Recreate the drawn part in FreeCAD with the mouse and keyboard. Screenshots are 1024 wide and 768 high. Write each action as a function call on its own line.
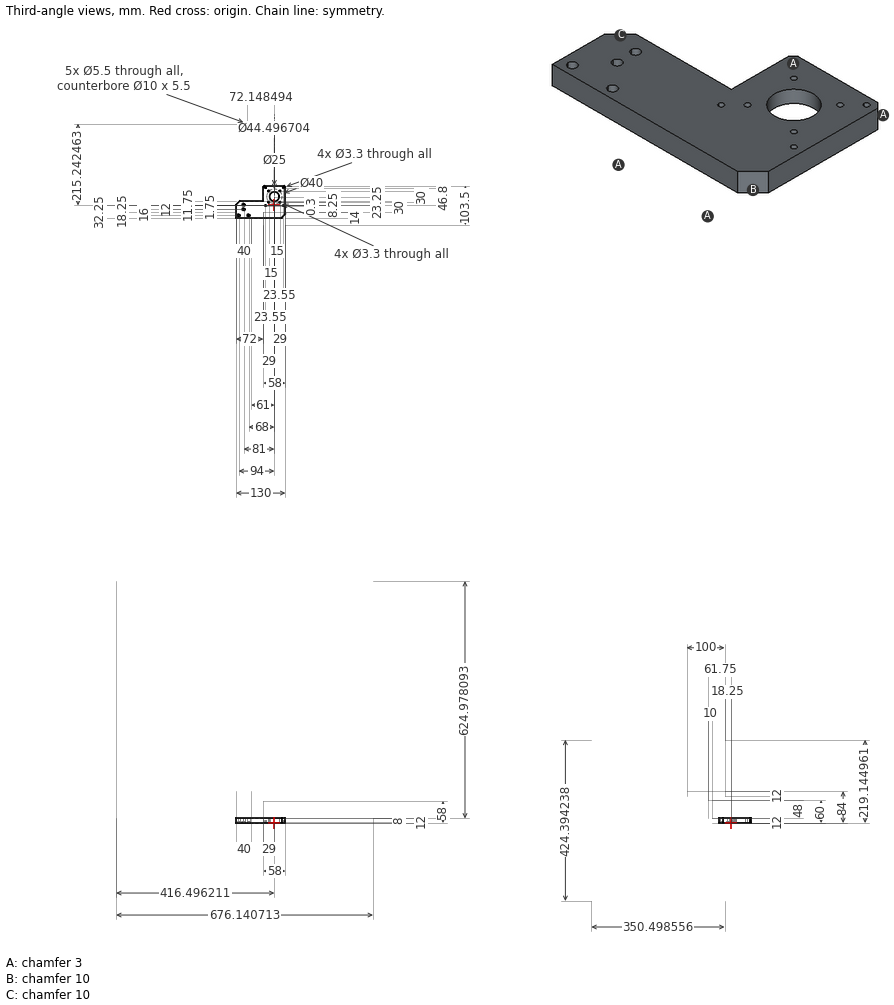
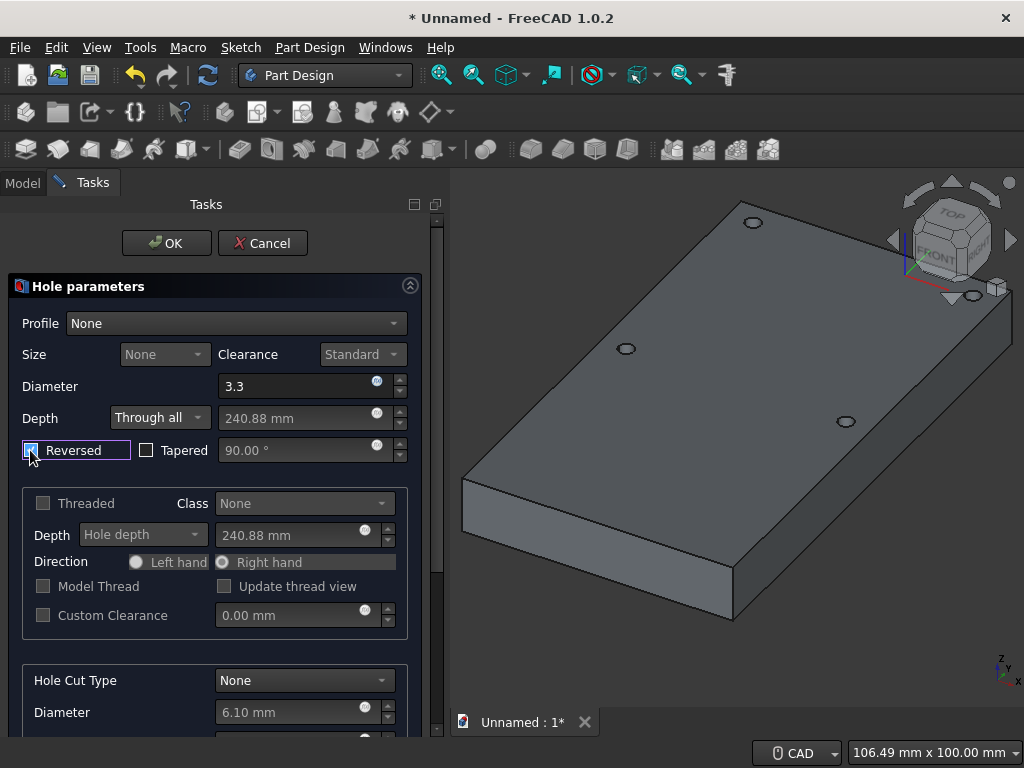
click(167, 243)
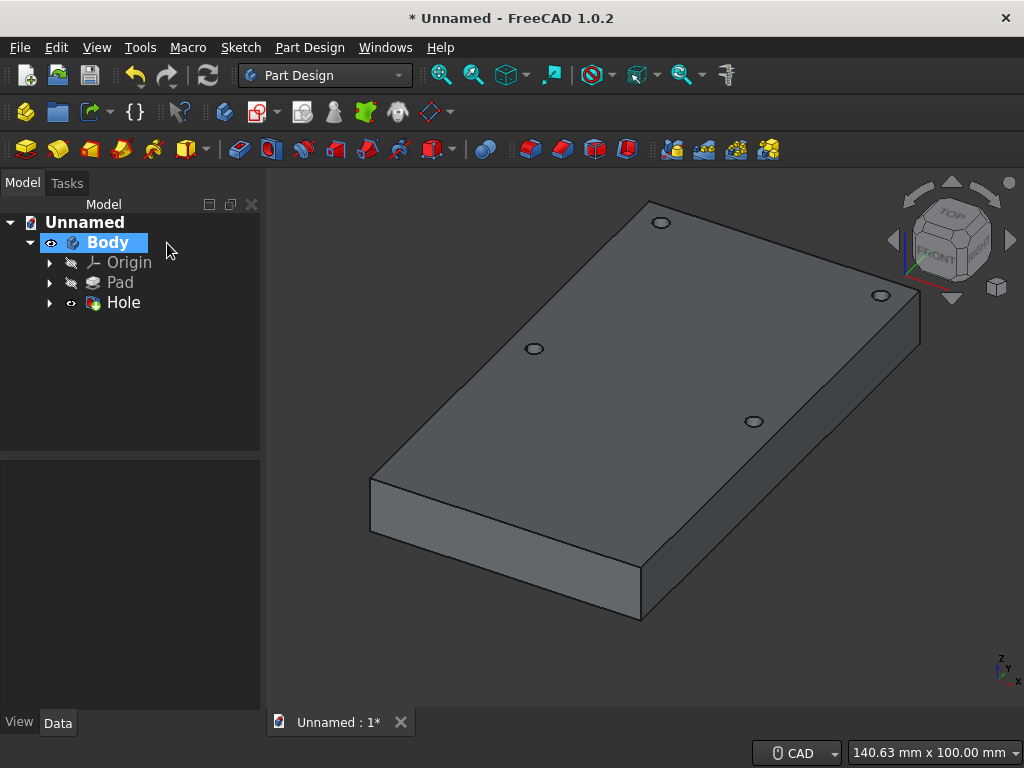
key(5)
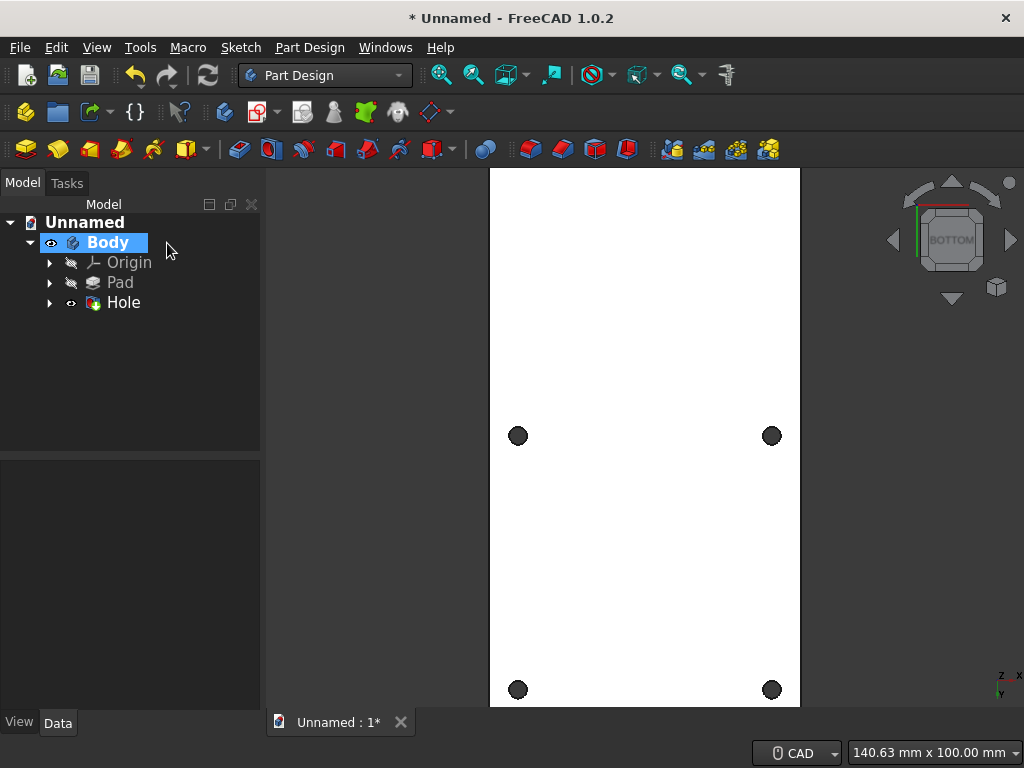
click(442, 76)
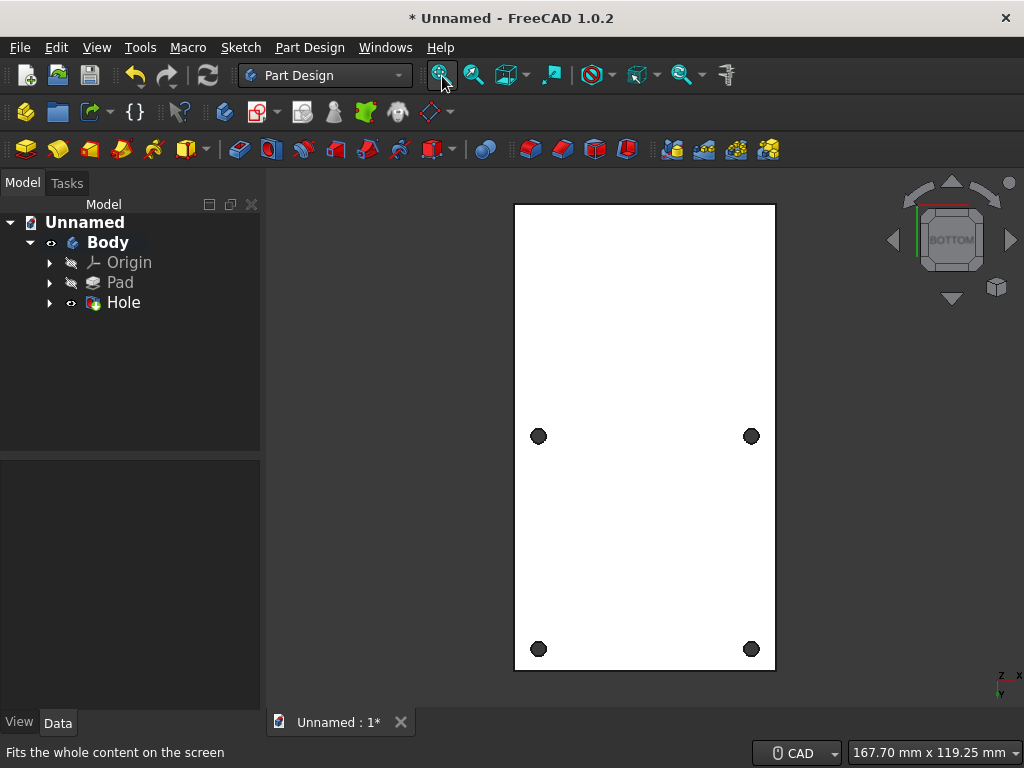
click(645, 503)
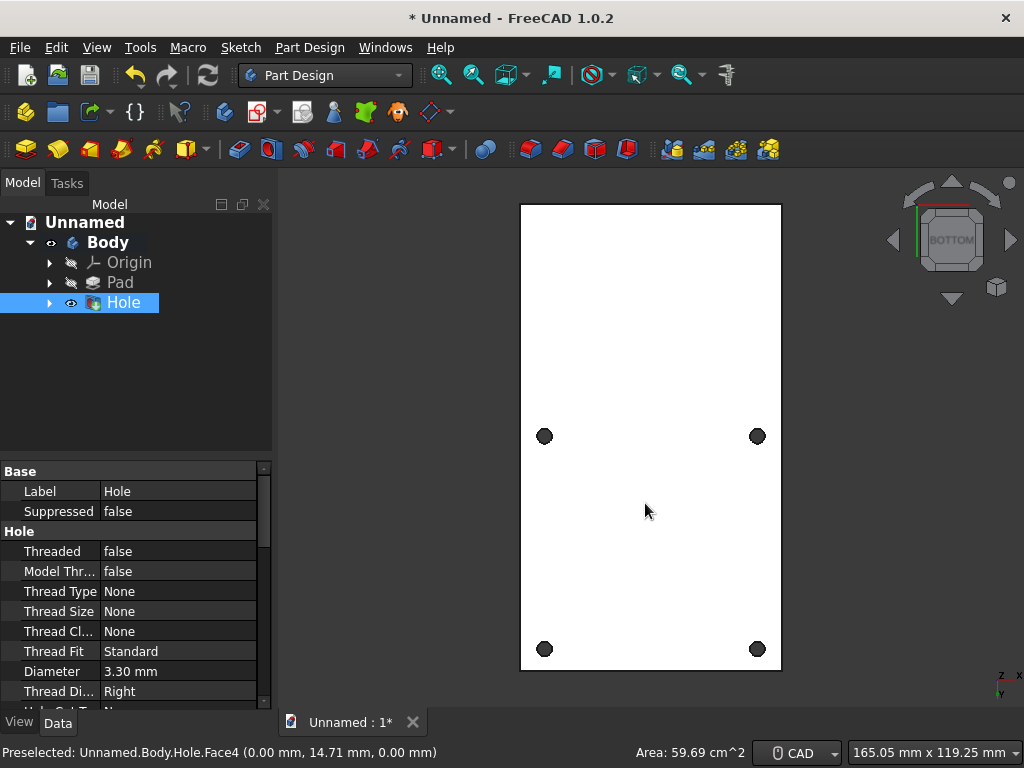
click(258, 112)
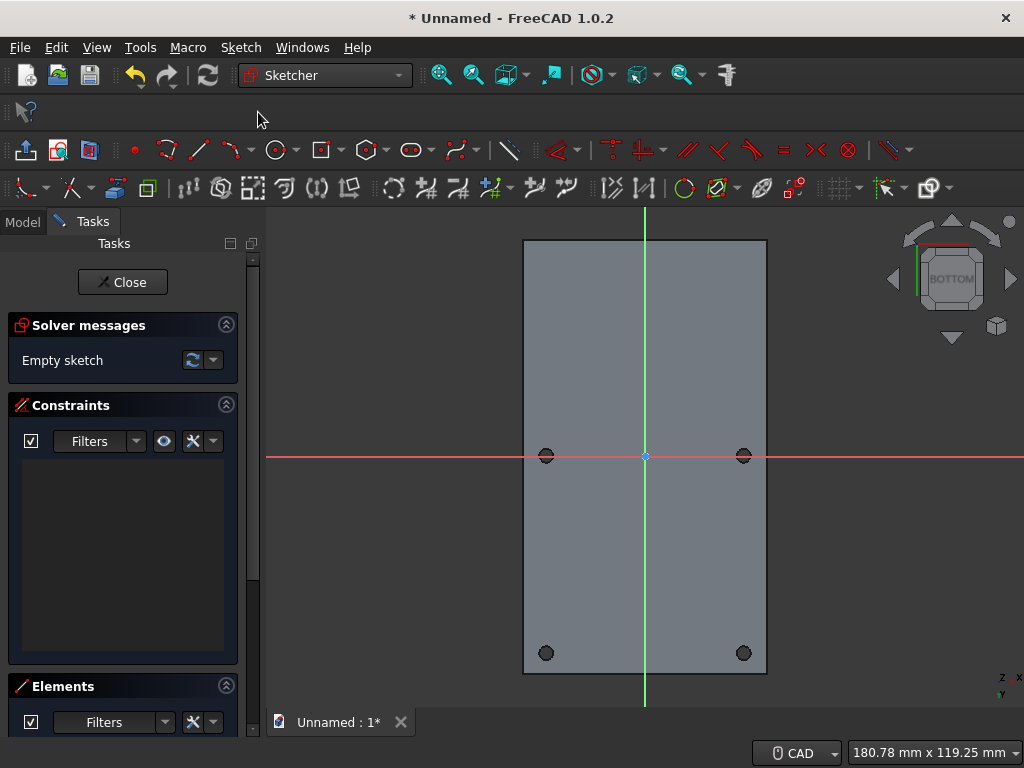
scroll(728, 658, up, 3)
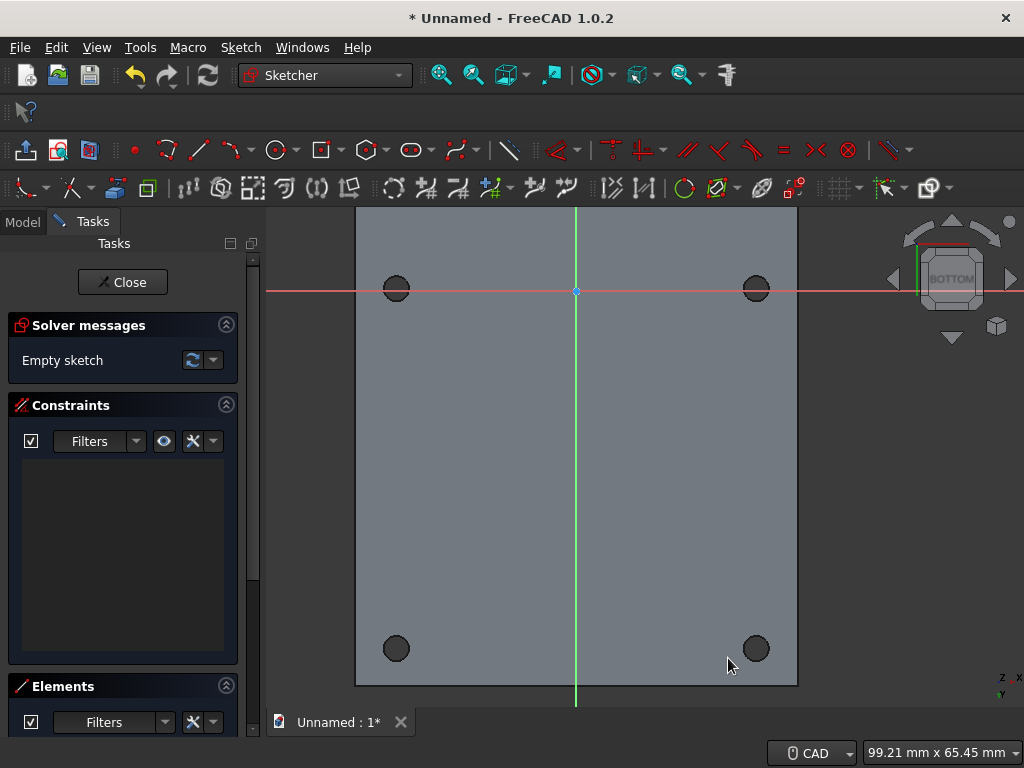
click(276, 150)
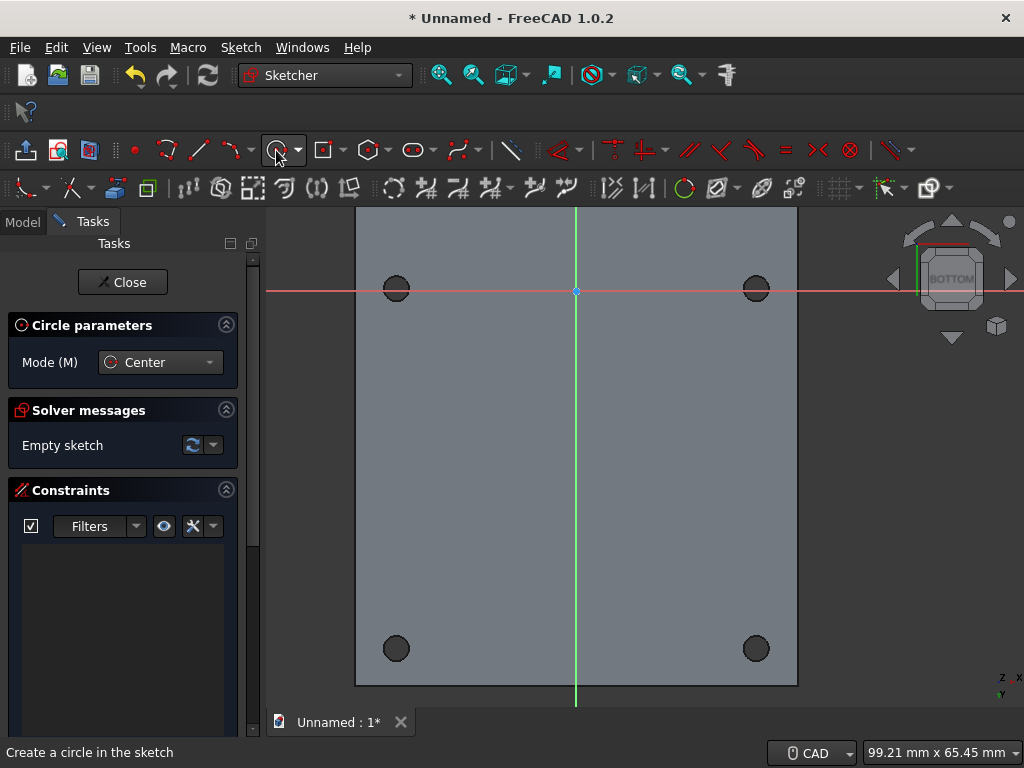
click(576, 469)
move(684, 361)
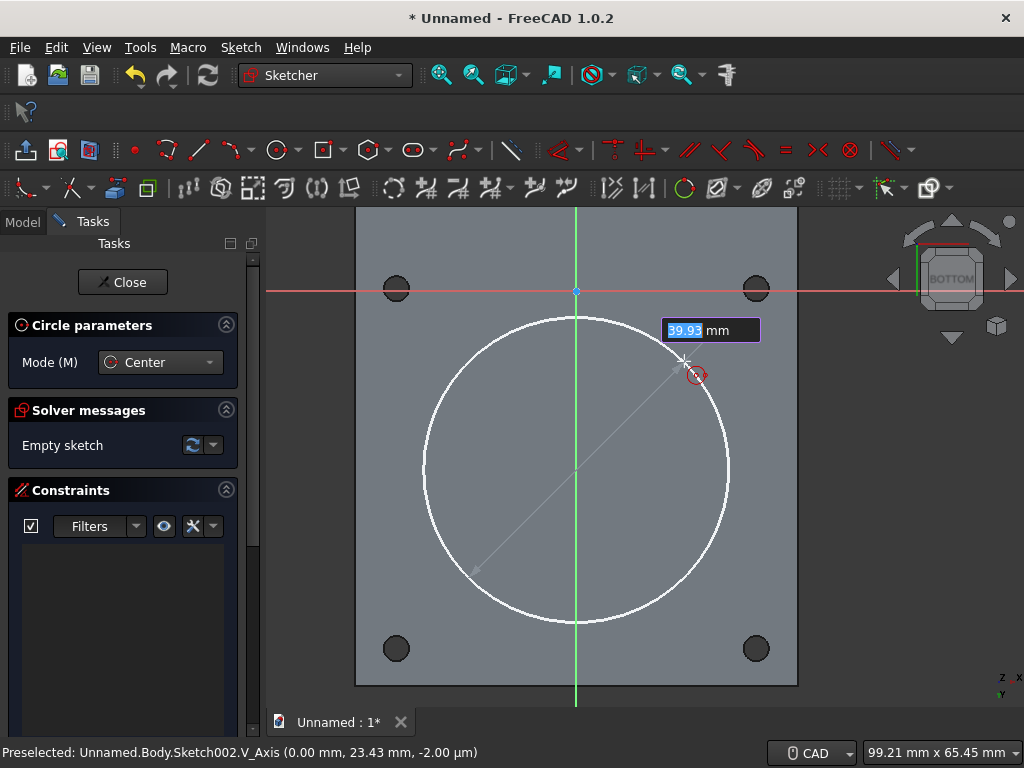
text(40)
key(Return)
key(Escape)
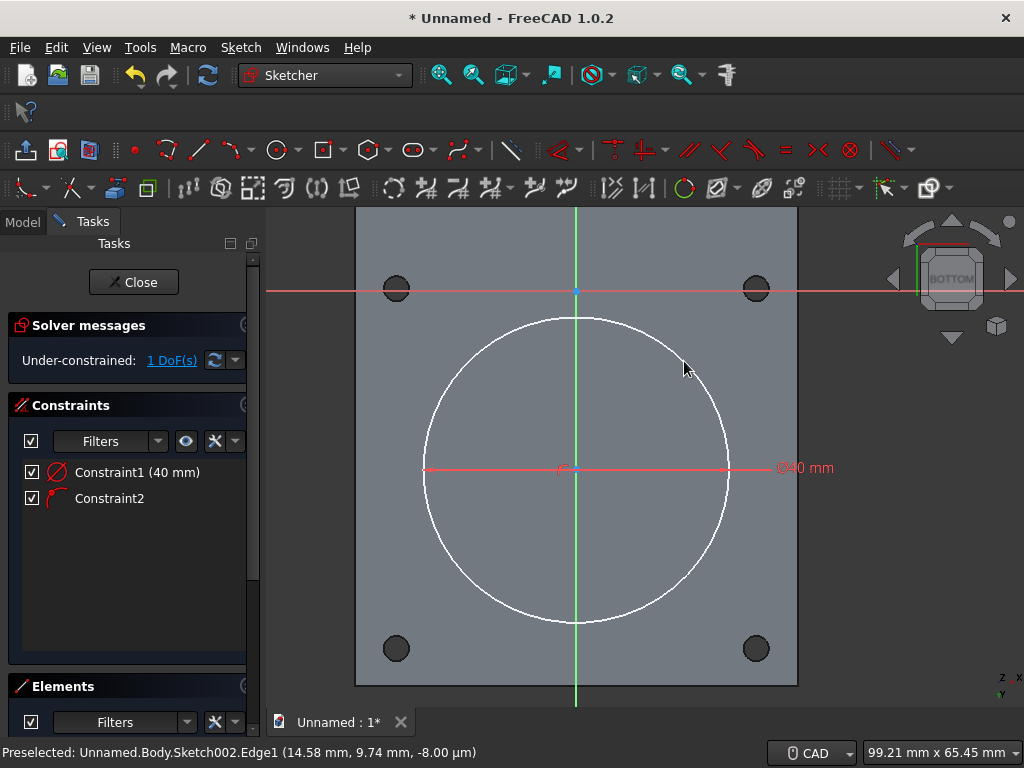
click(558, 150)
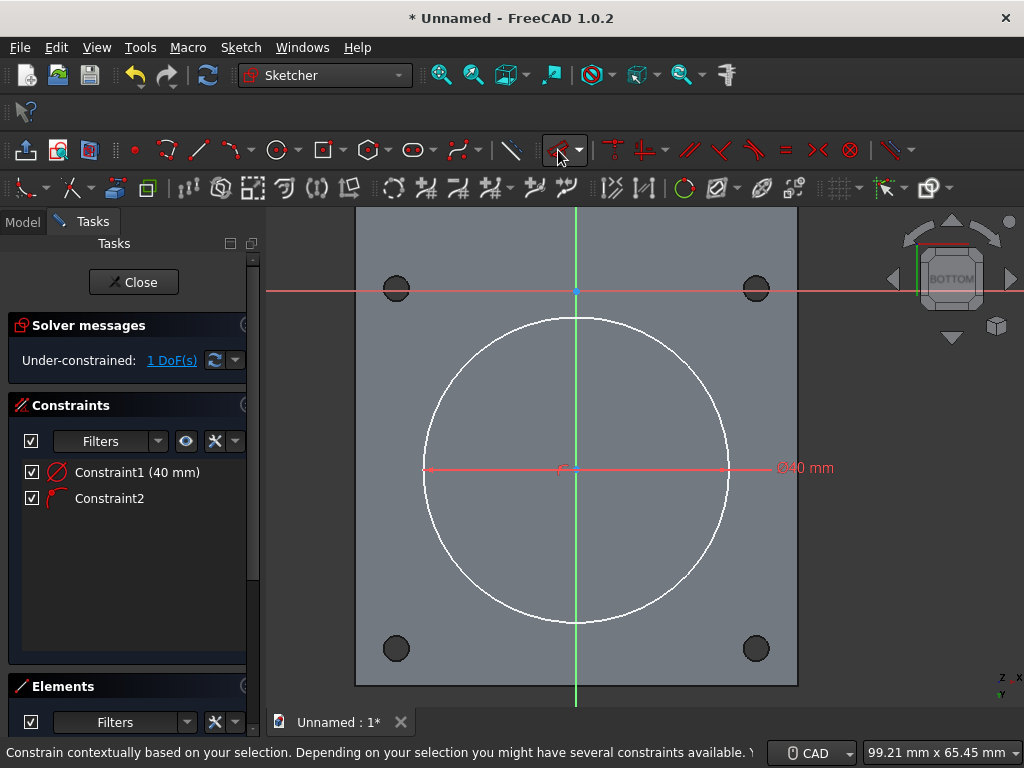
click(576, 470)
click(610, 381)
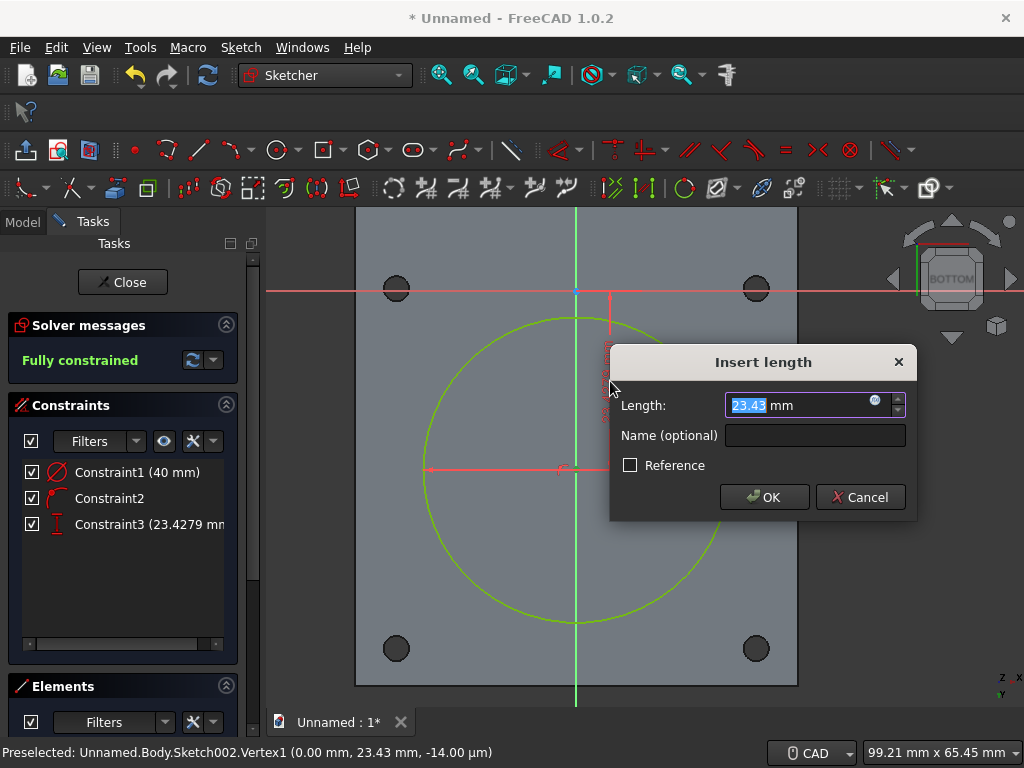
text(23.25)
key(Return)
key(Escape)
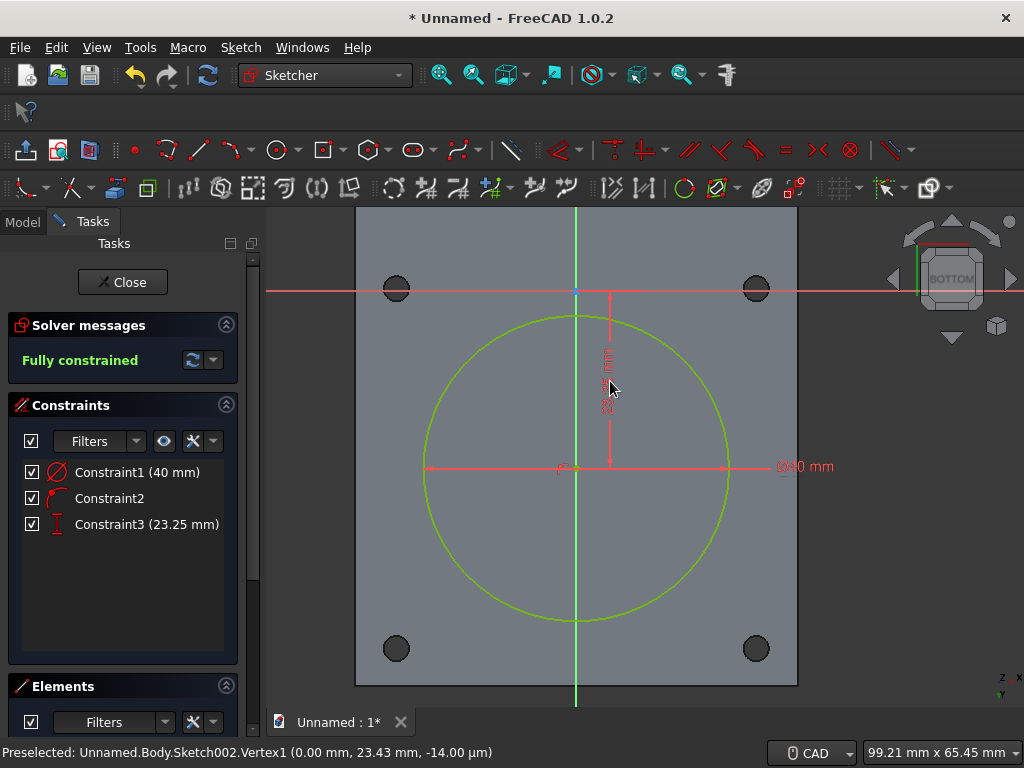
click(123, 282)